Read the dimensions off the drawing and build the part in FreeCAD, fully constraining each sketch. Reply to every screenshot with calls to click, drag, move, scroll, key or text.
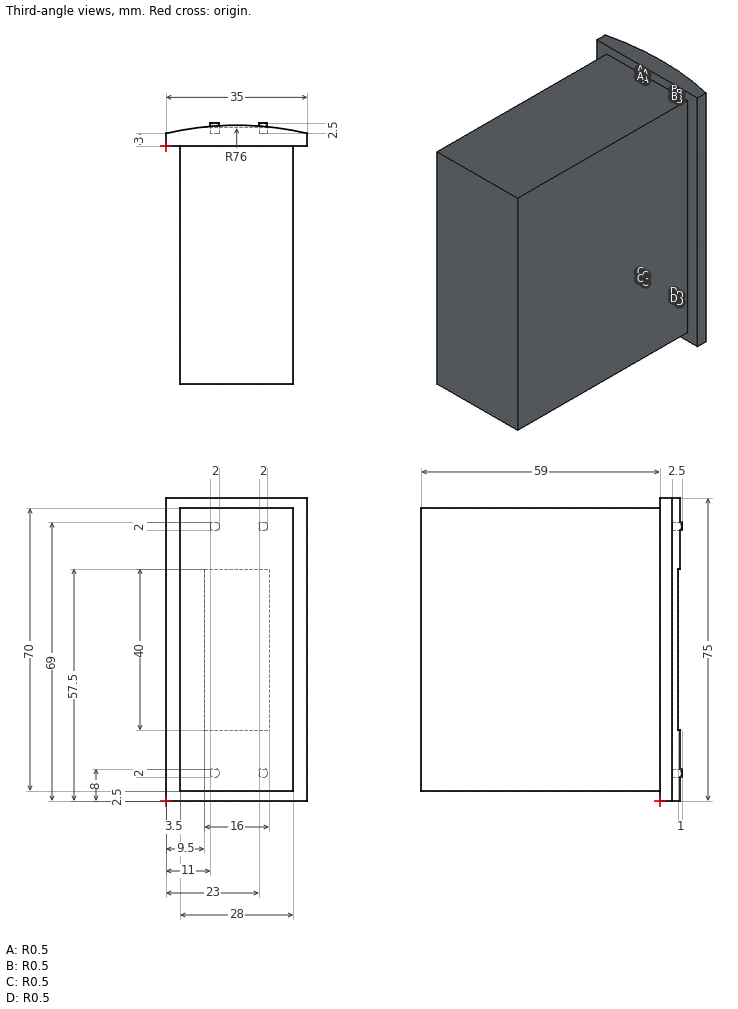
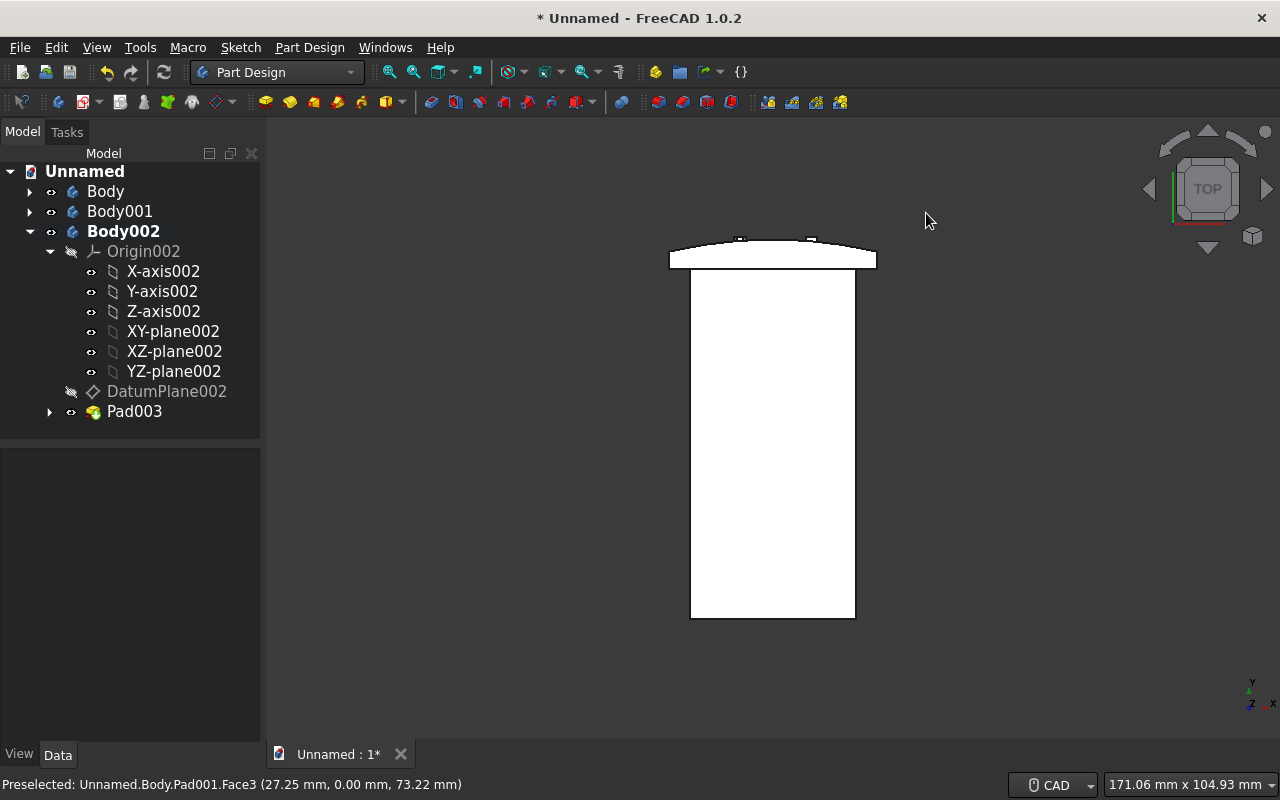
click(390, 72)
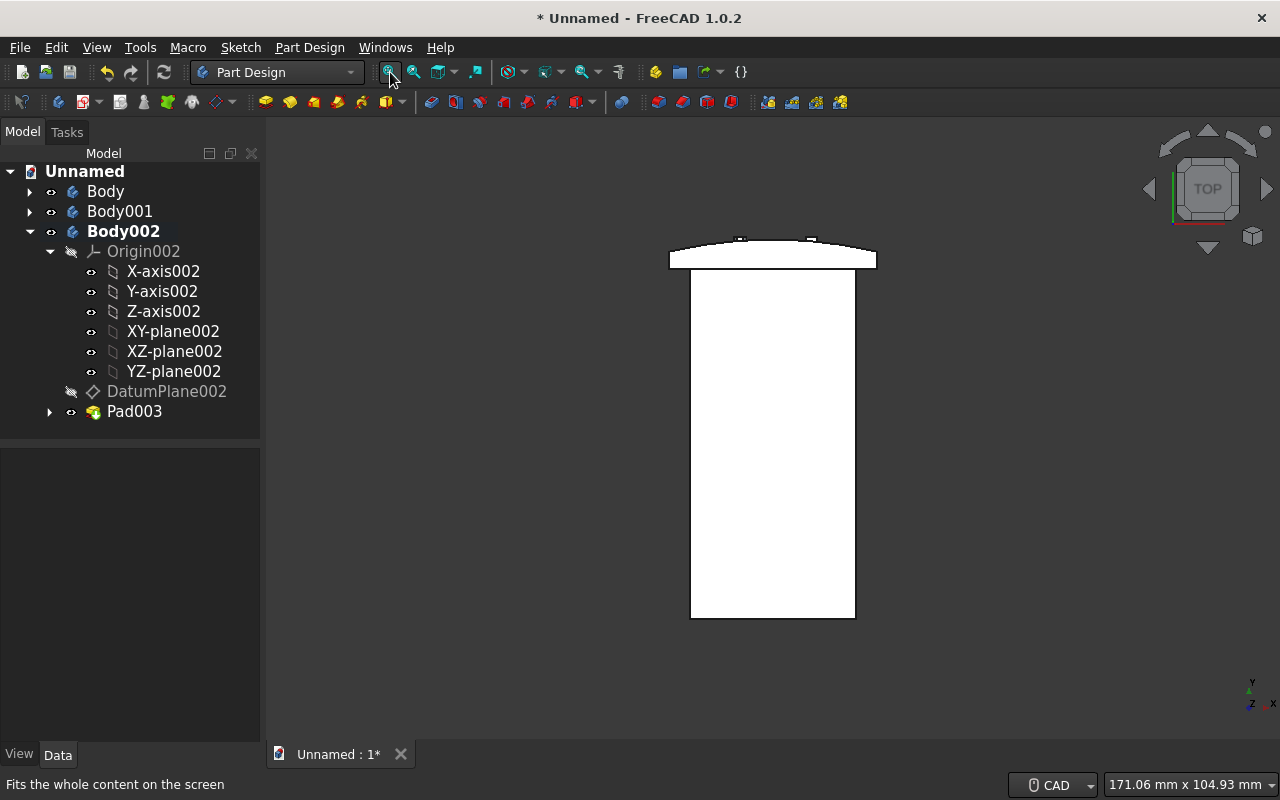
scroll(806, 243, up, 5)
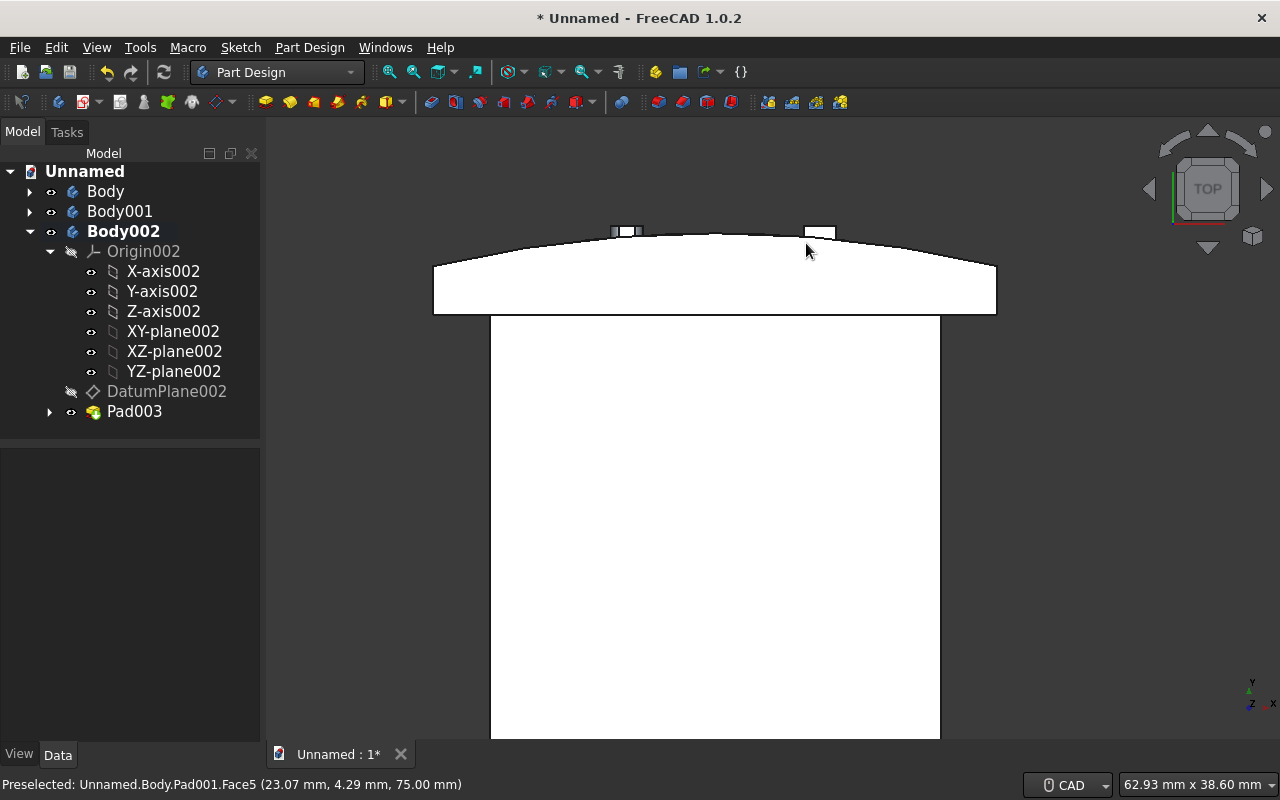
key(v)
key(f)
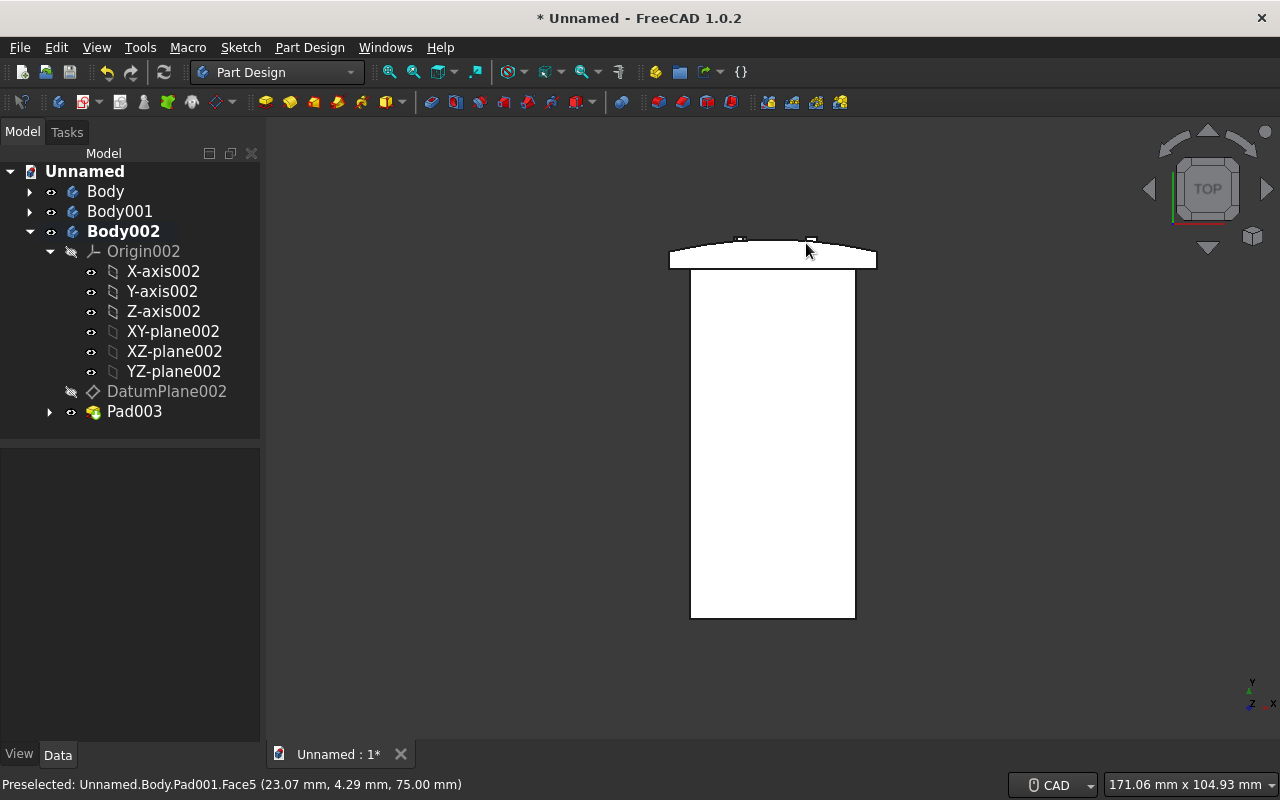
key(0)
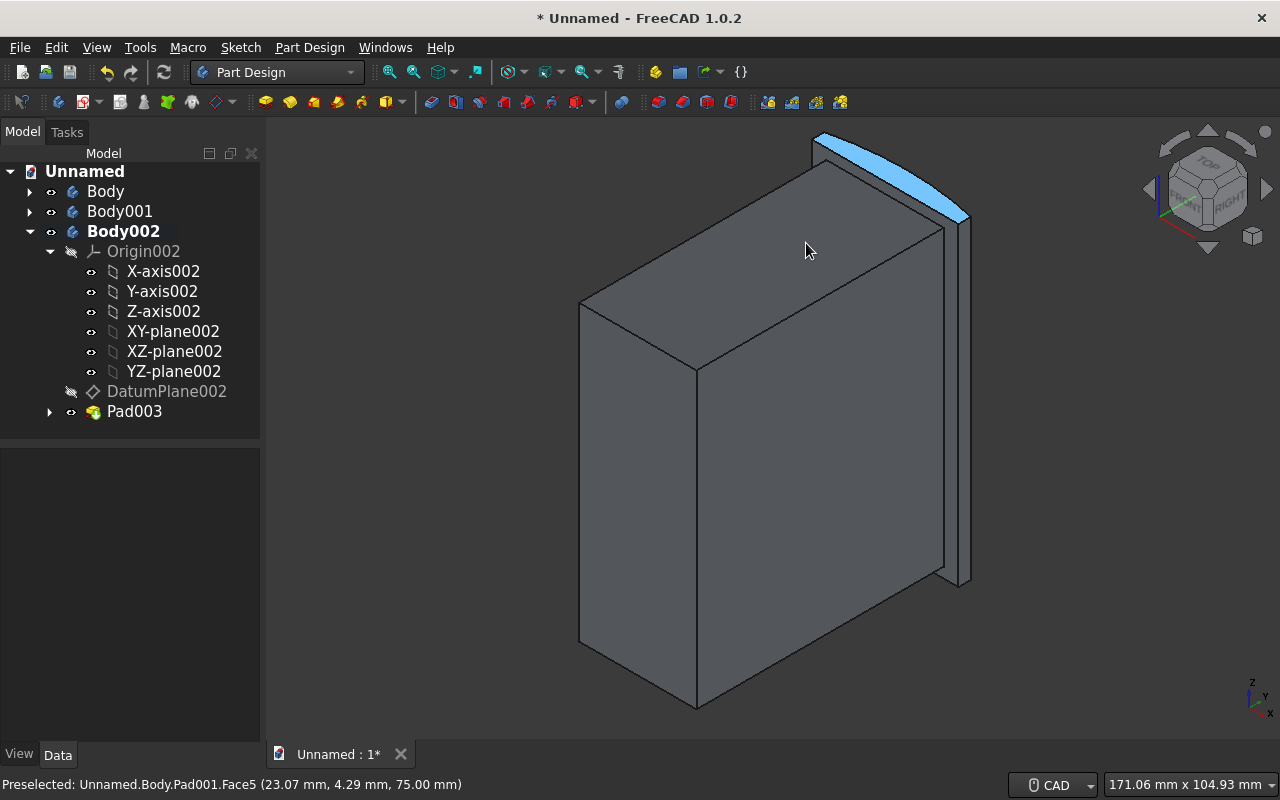
click(390, 72)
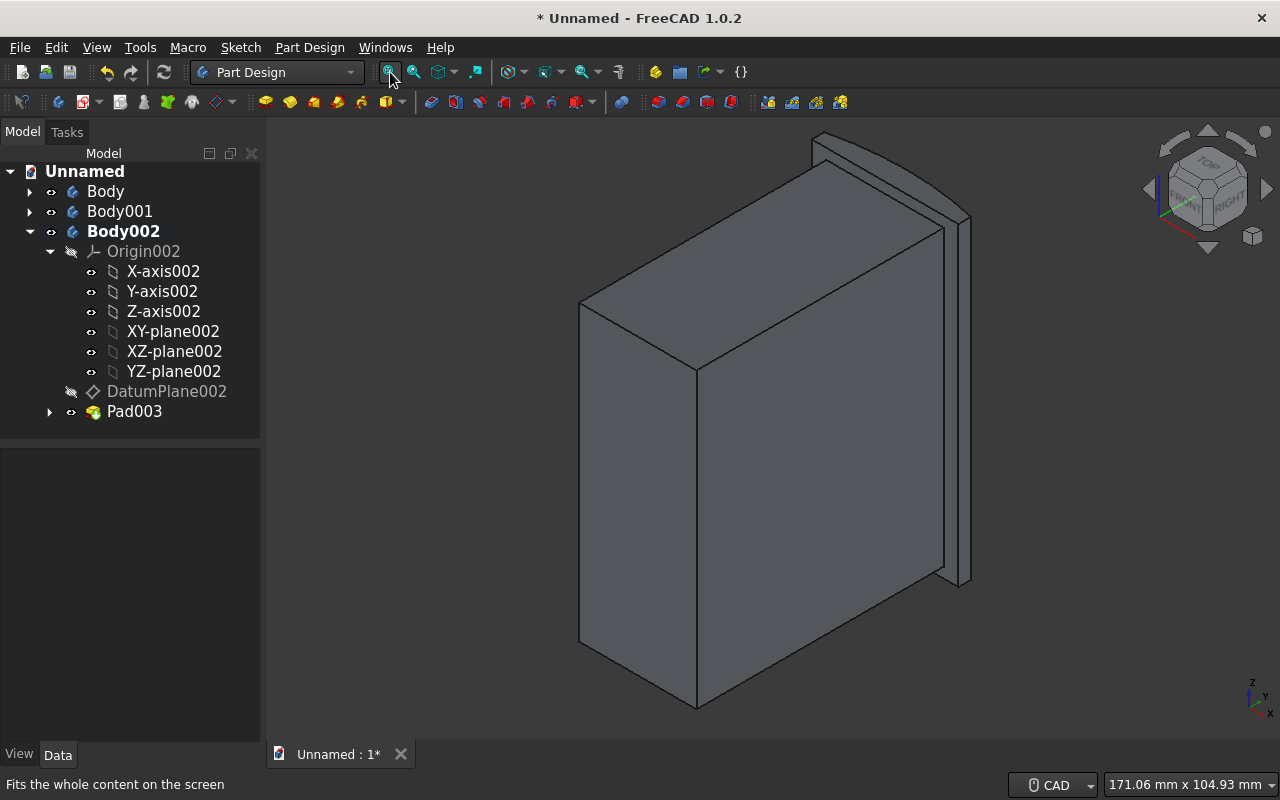
scroll(926, 213, up, 5)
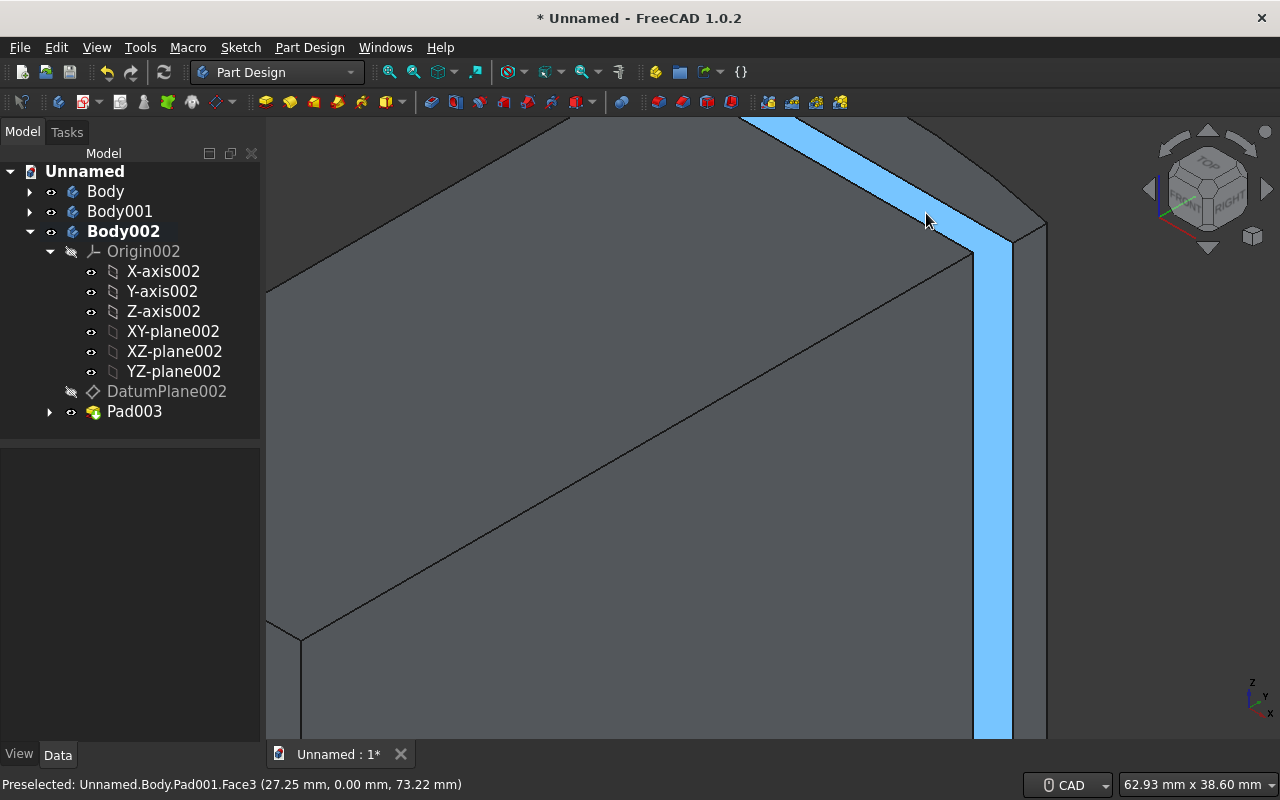
click(390, 72)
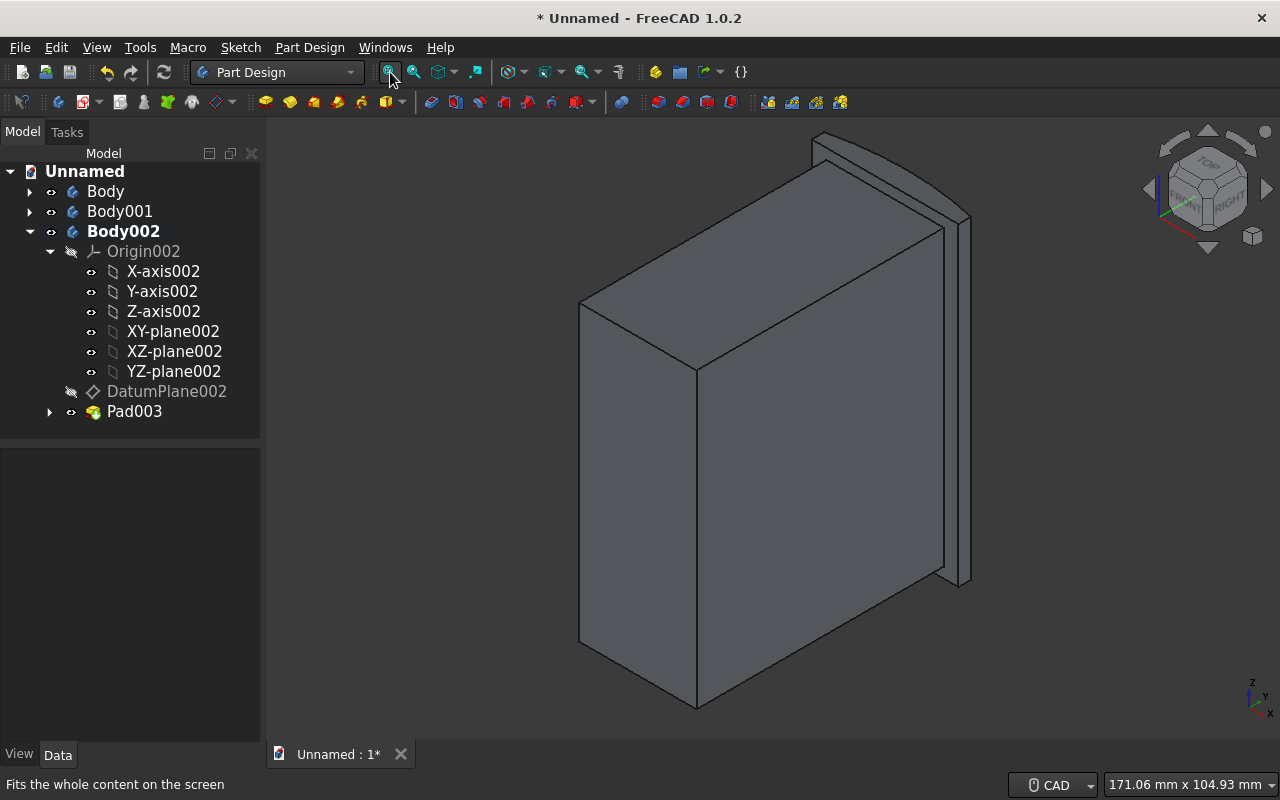
key(1)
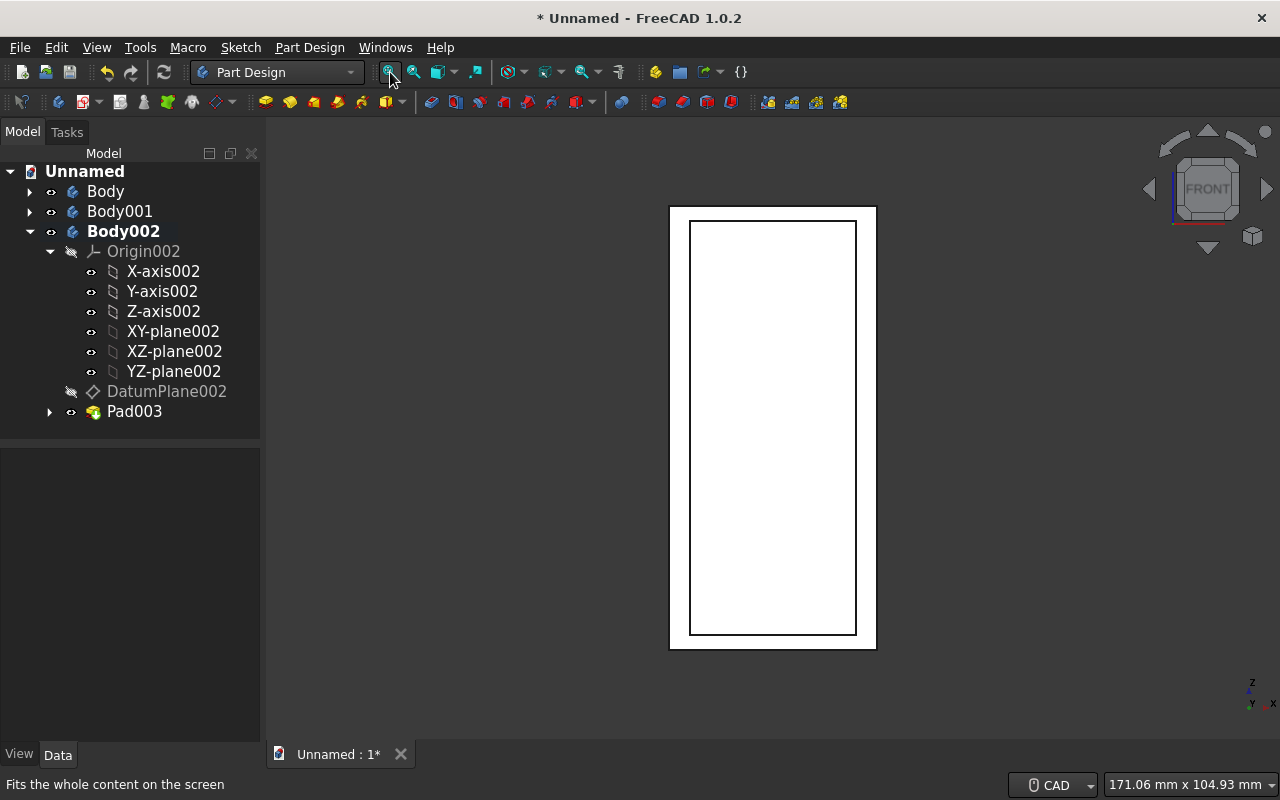
key(v)
key(f)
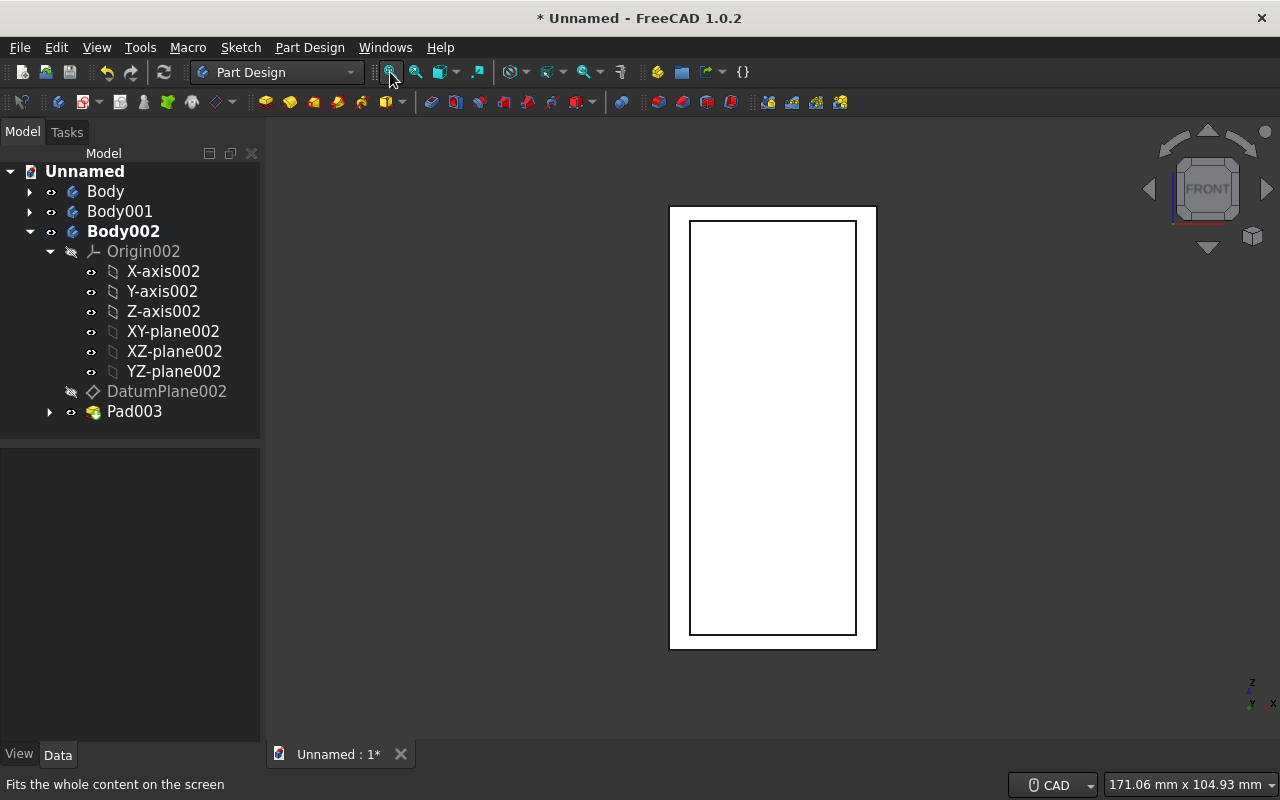
scroll(806, 240, up, 5)